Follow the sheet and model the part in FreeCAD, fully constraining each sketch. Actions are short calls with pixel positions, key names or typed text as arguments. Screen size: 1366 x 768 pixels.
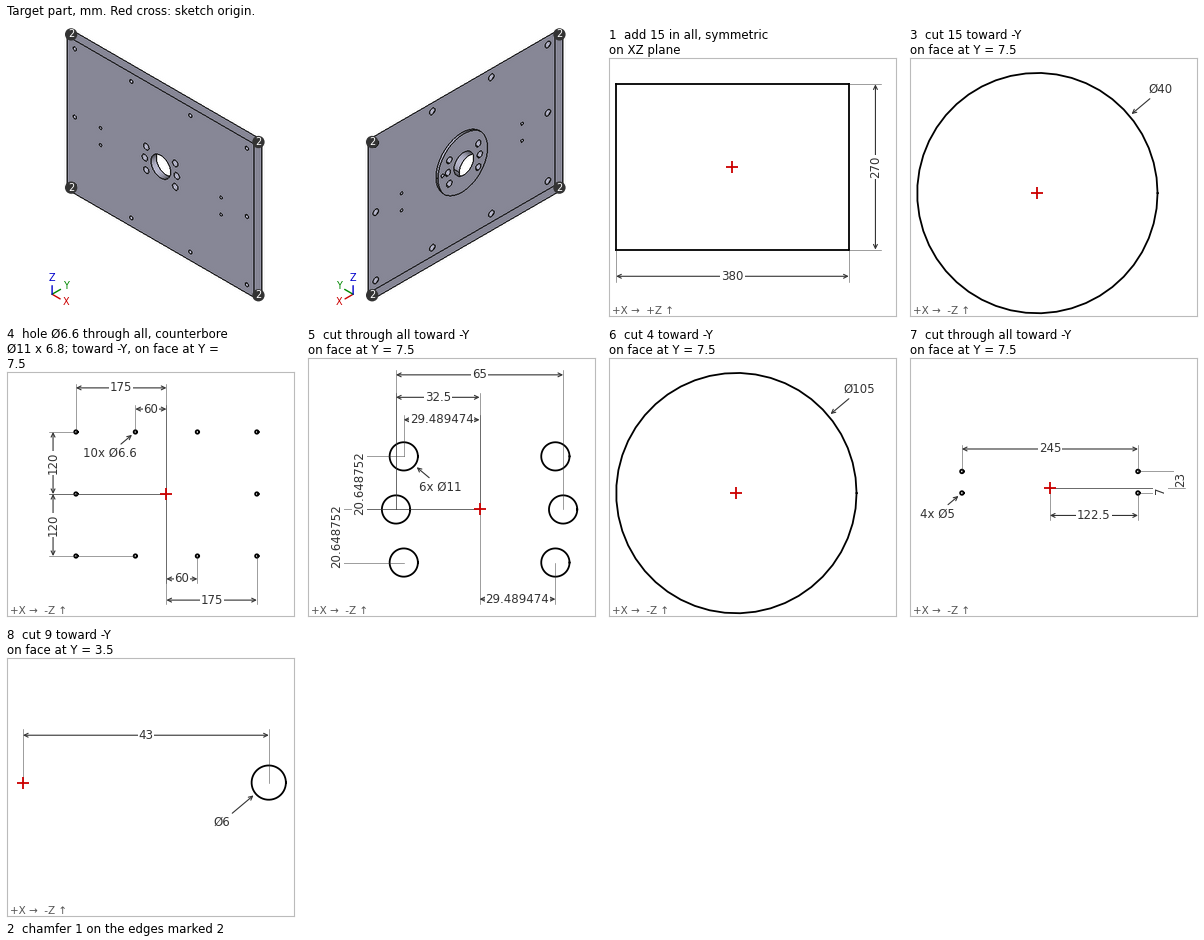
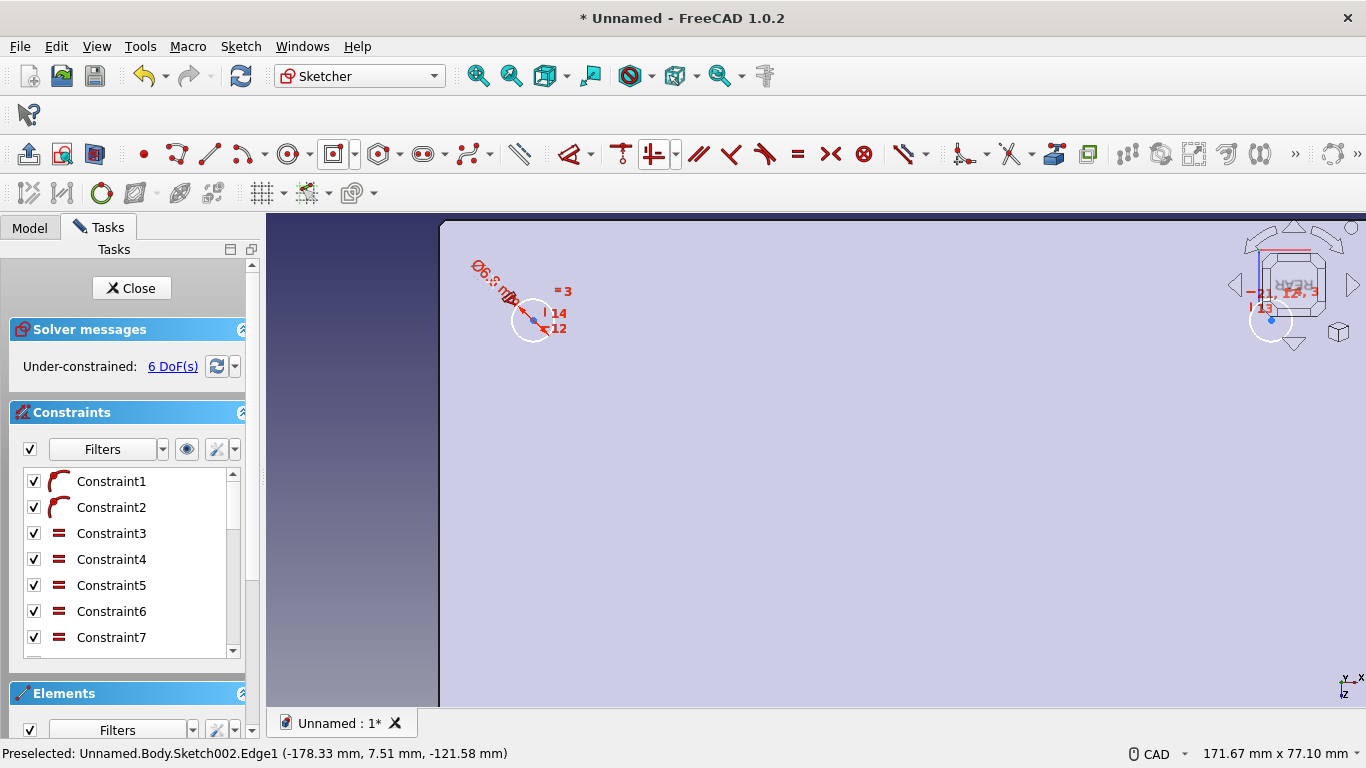
scroll(518, 302, down, 8)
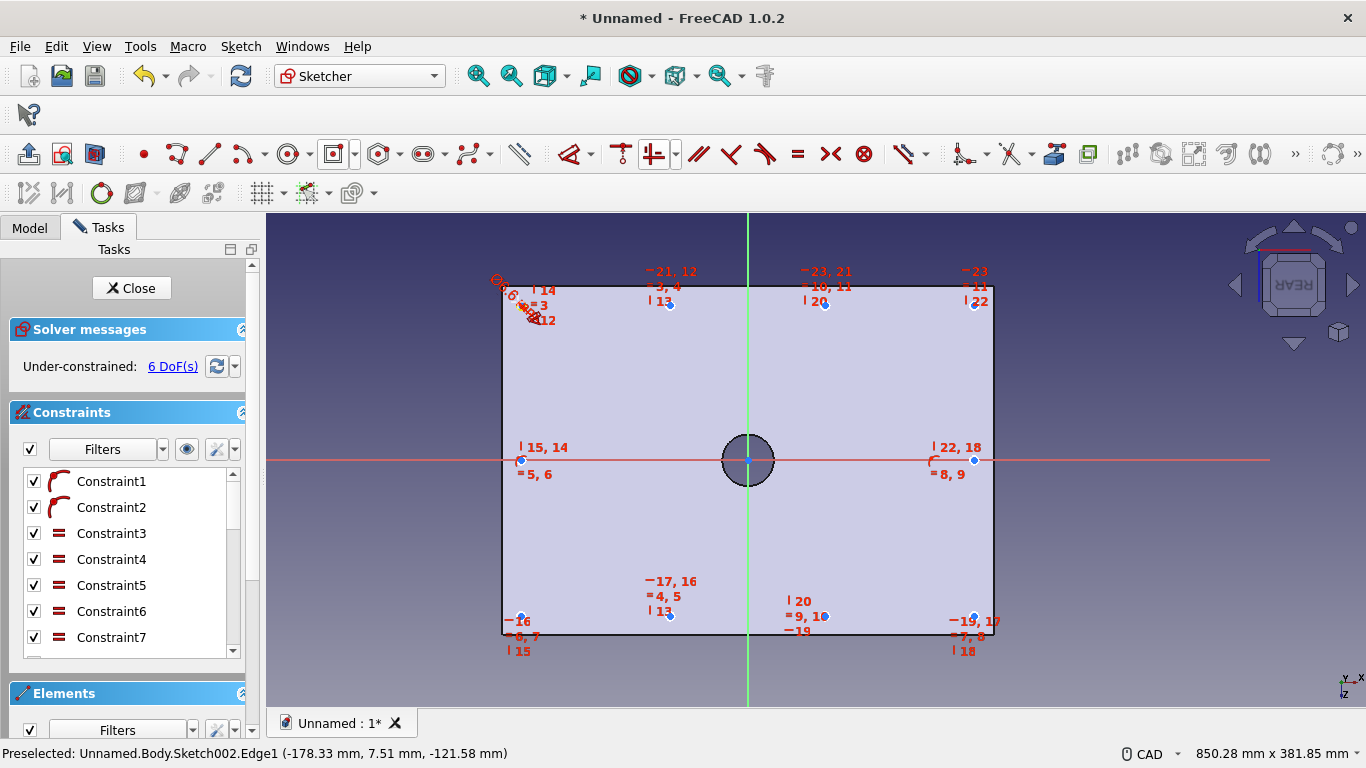
click(670, 306)
click(709, 272)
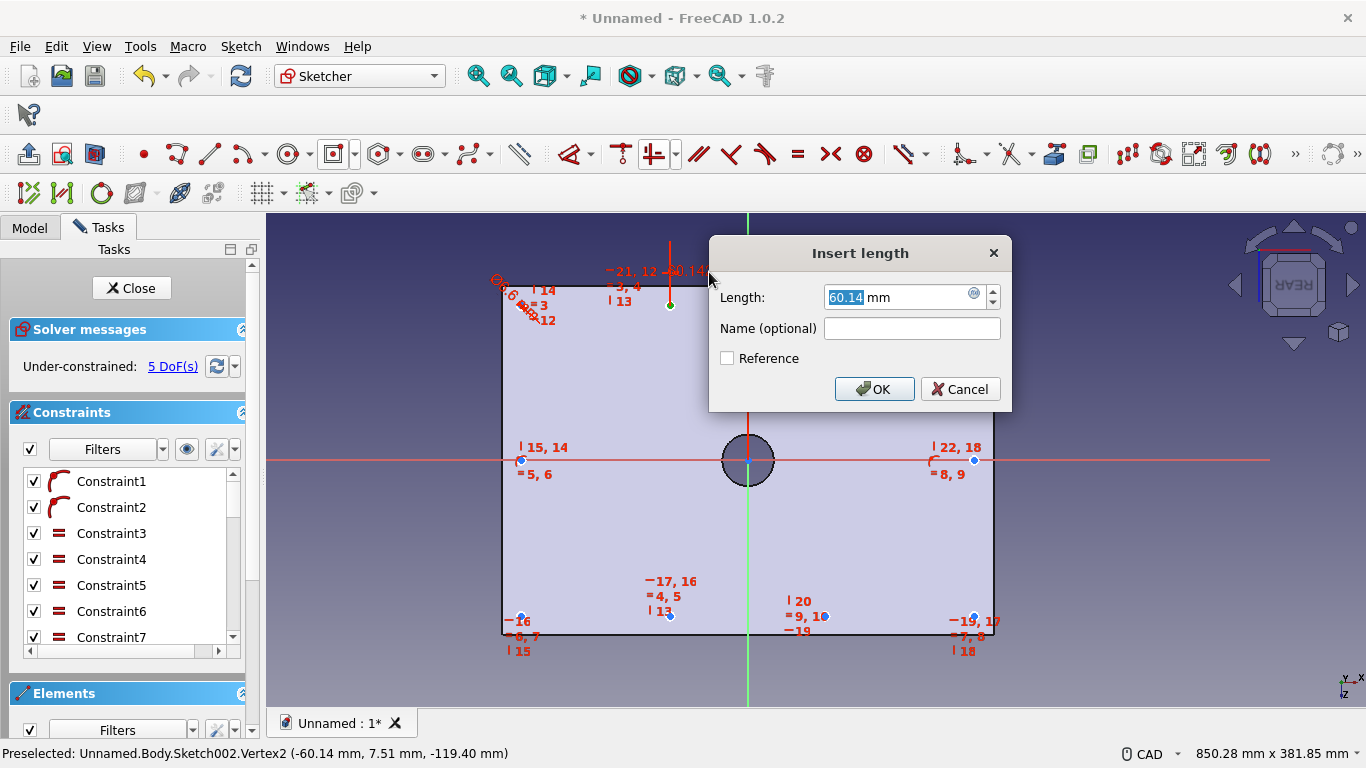
text(60)
key(Return)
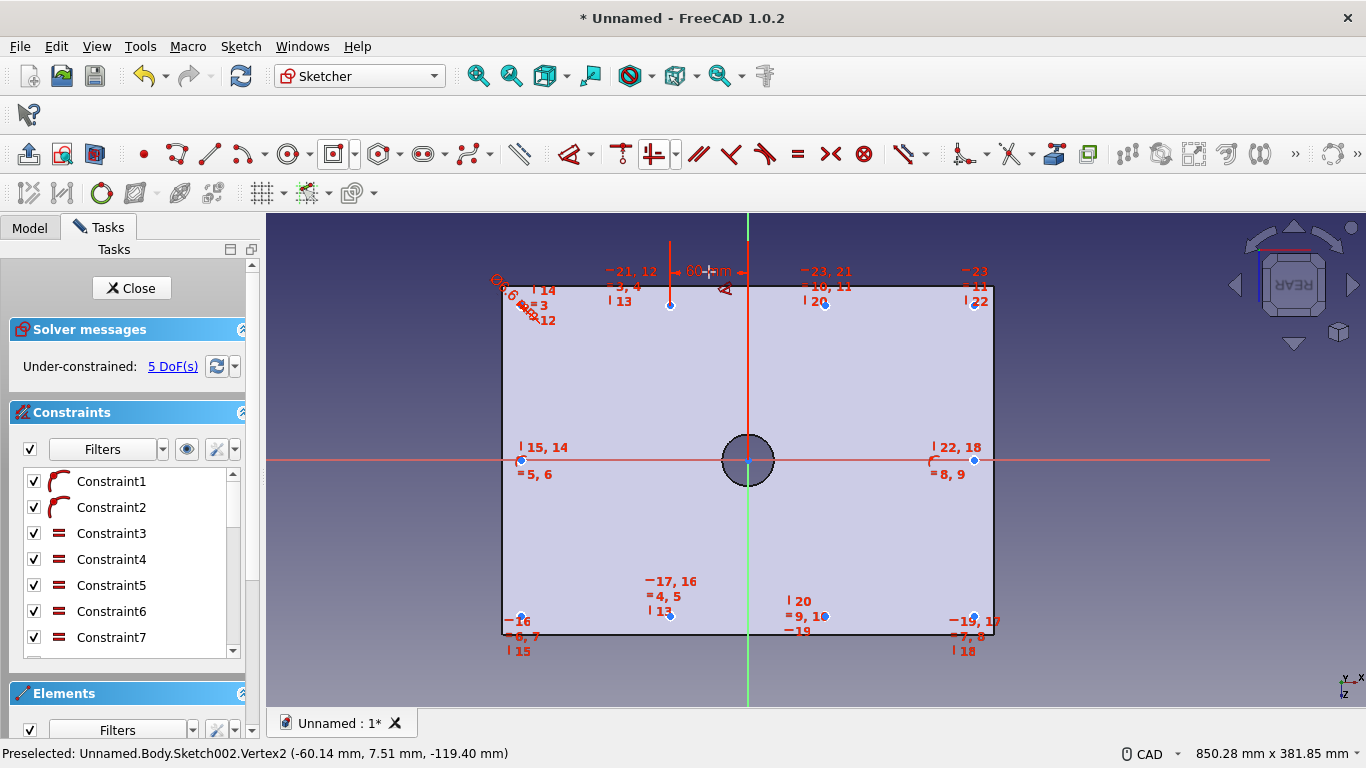
click(825, 616)
click(787, 650)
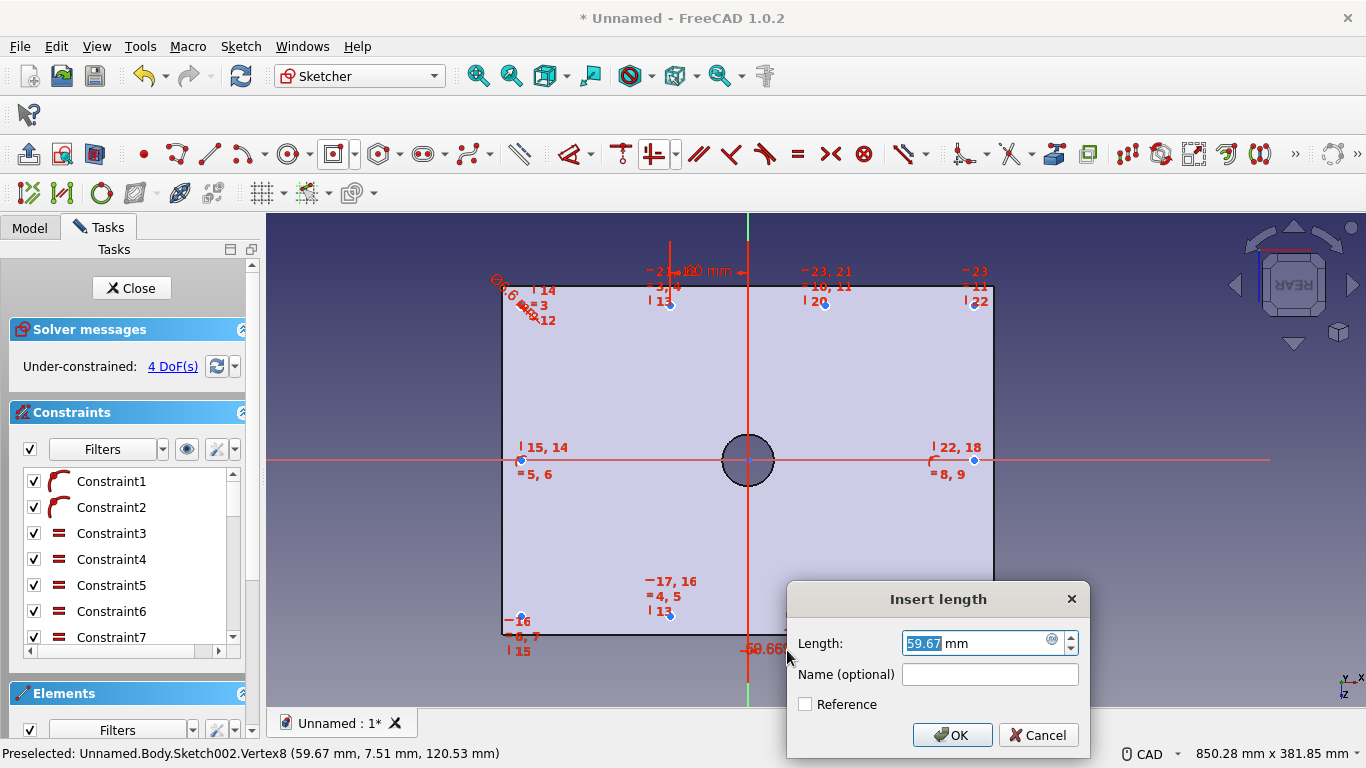
text(60)
key(Return)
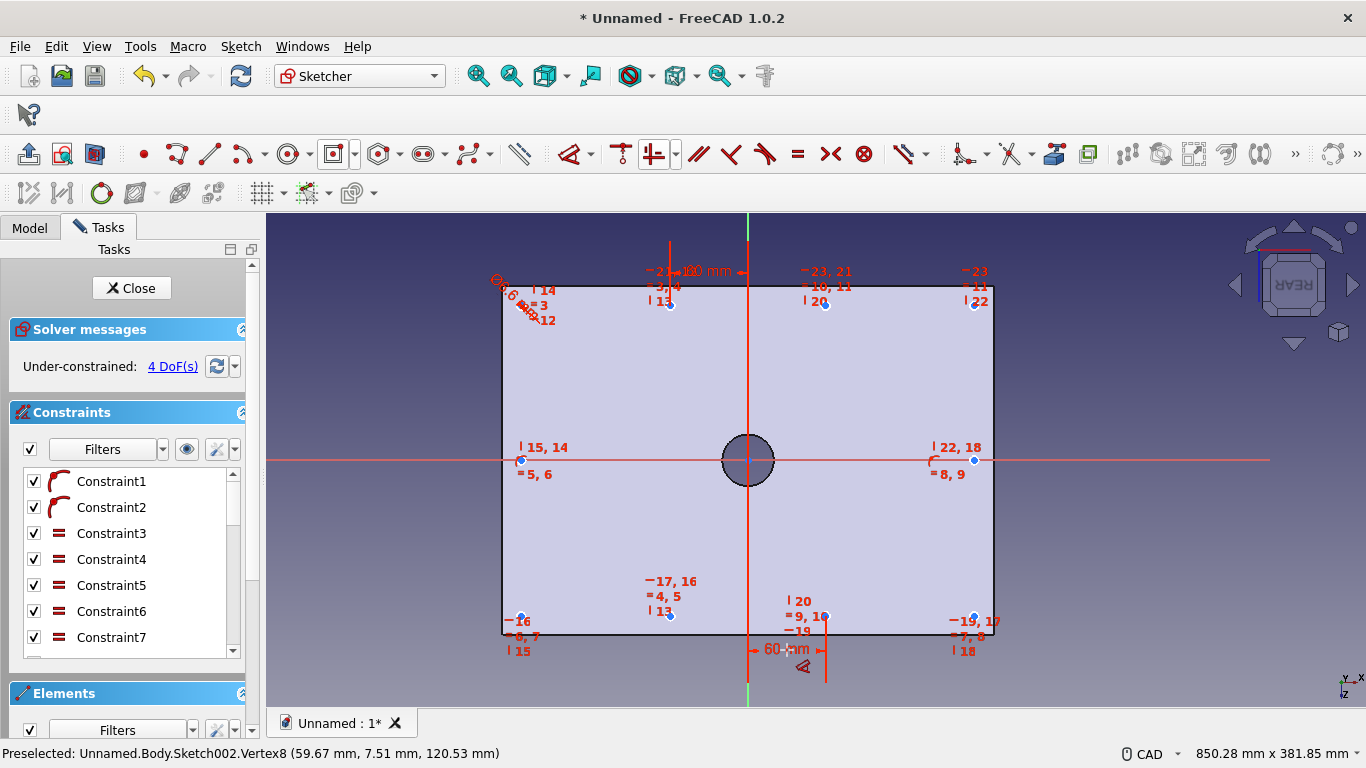
click(521, 306)
click(635, 272)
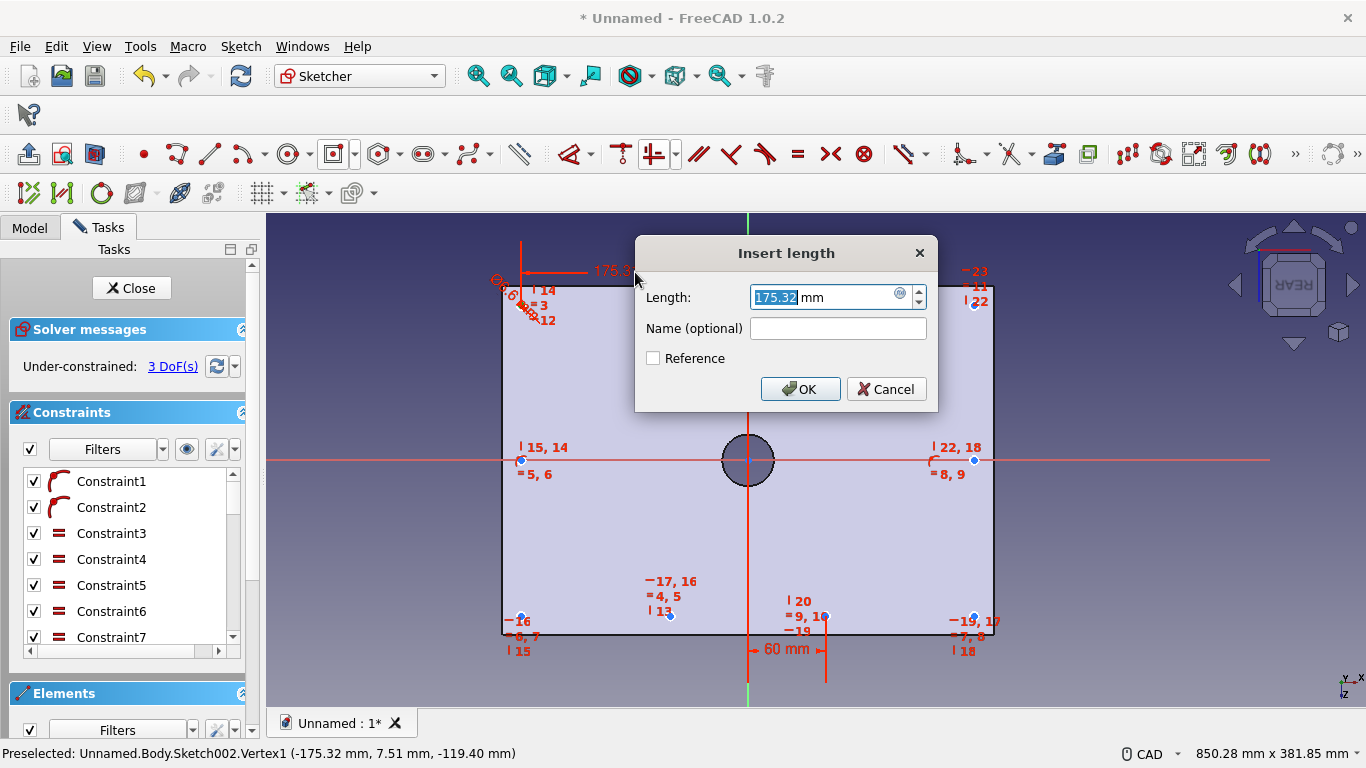
text(175)
key(Return)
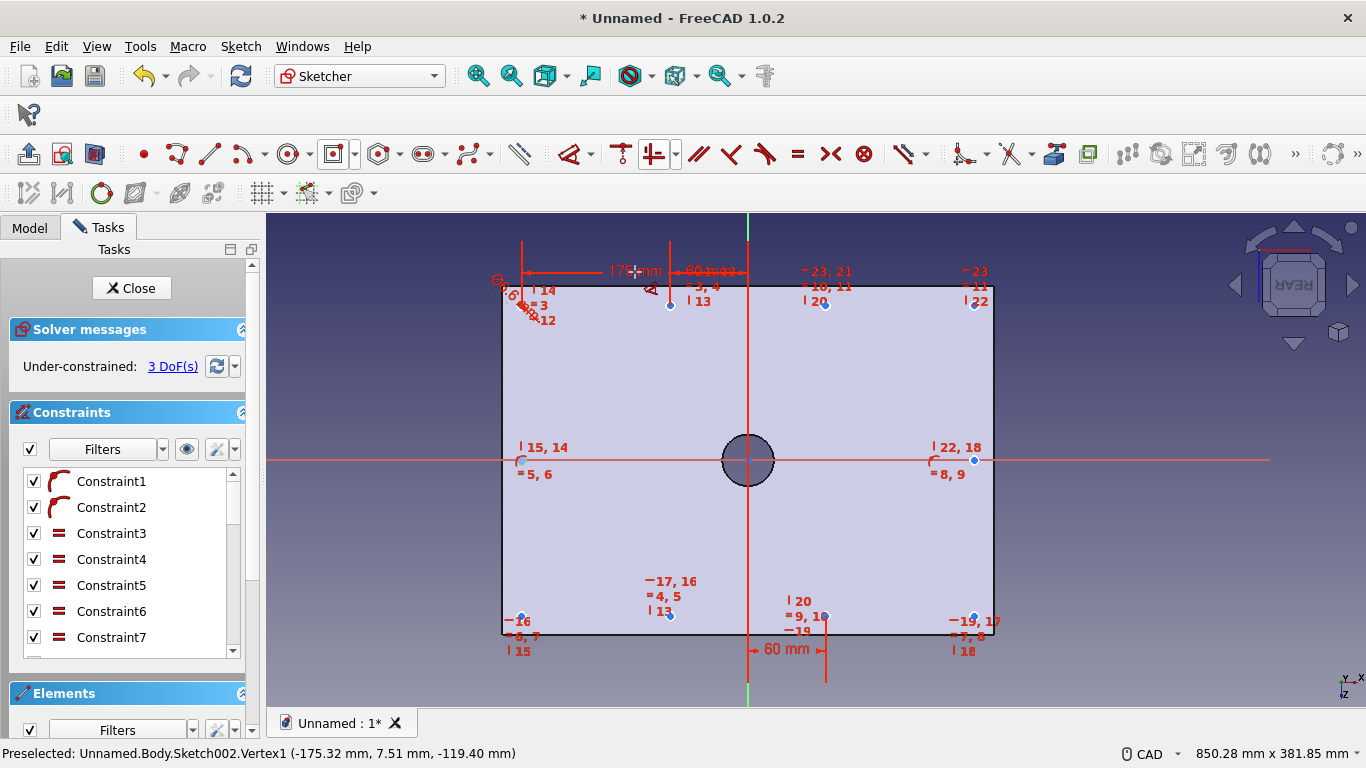
click(522, 306)
click(488, 383)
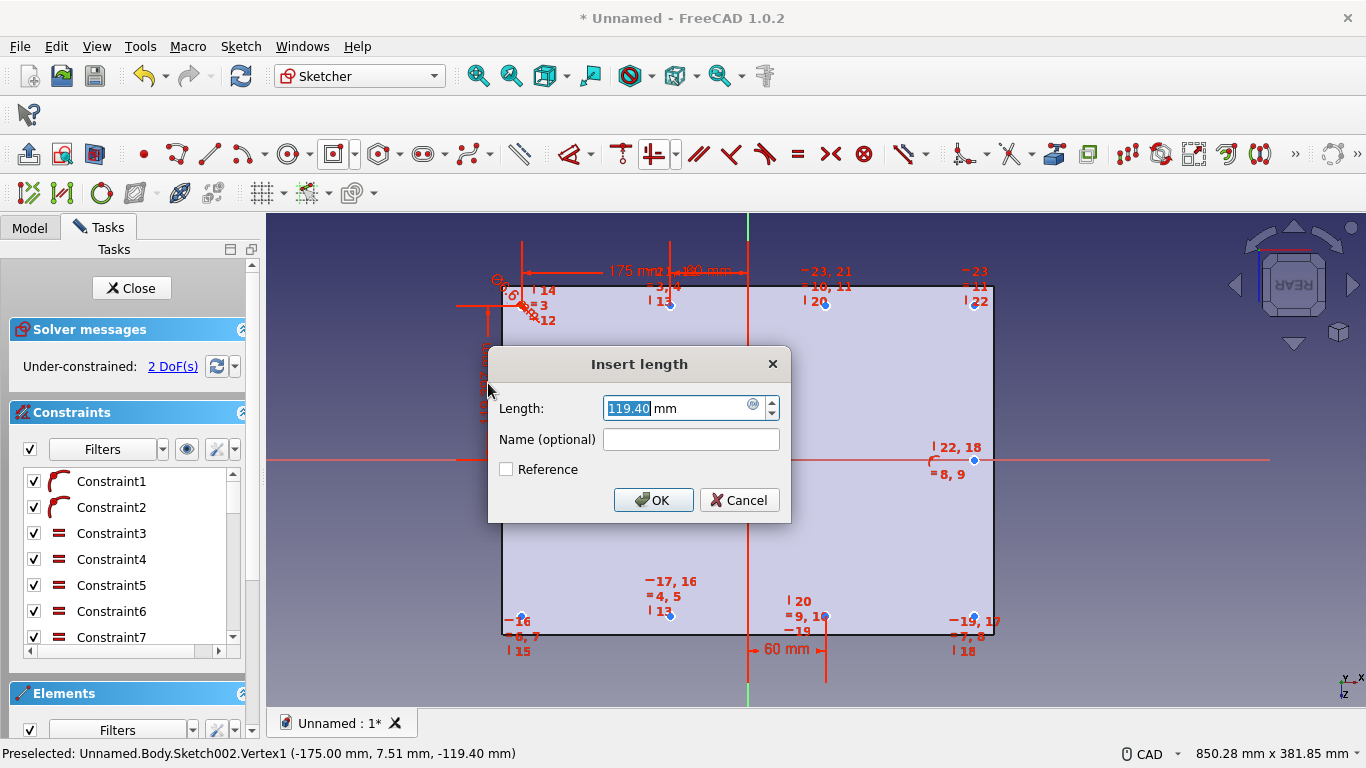
text(120)
key(Return)